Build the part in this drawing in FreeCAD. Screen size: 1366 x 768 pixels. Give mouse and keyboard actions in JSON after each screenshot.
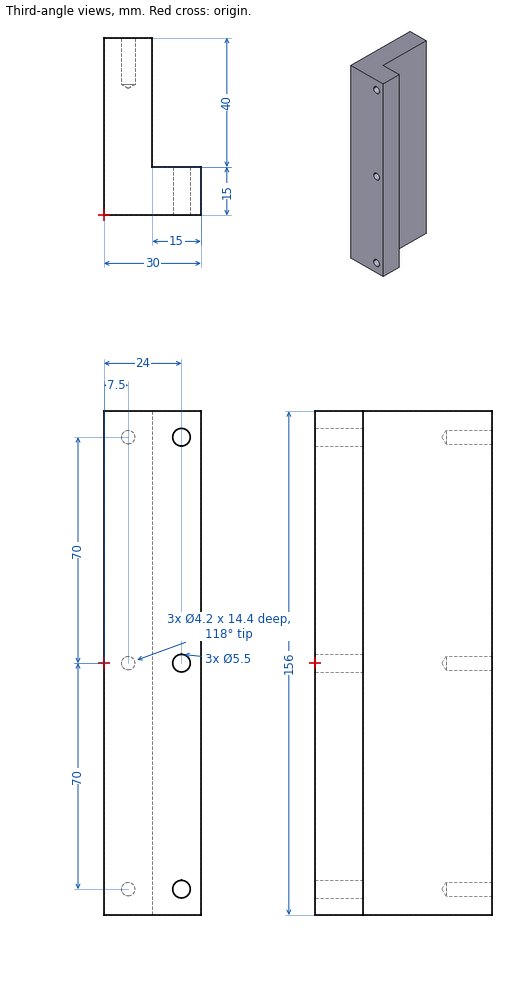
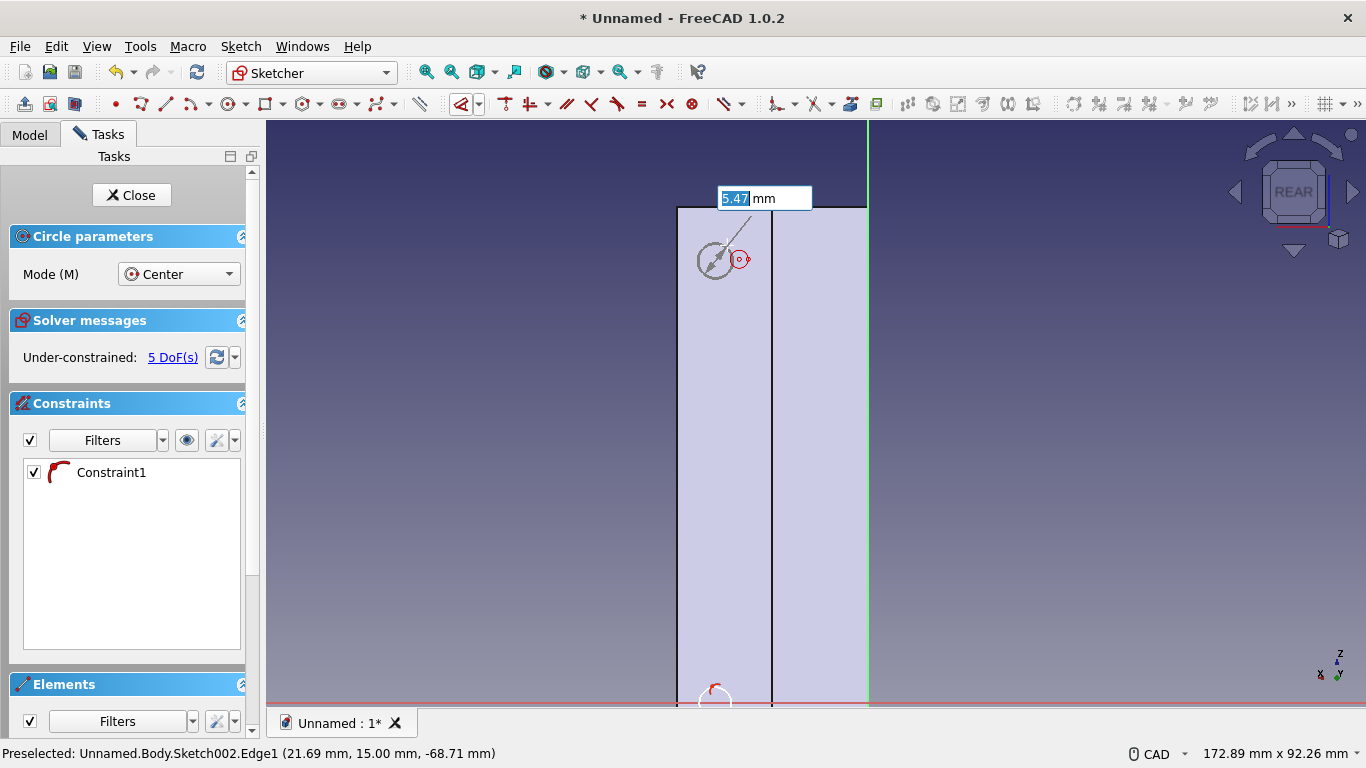
{"action": "left_click", "coordinate": [727, 246]}
{"action": "key", "text": "Escape"}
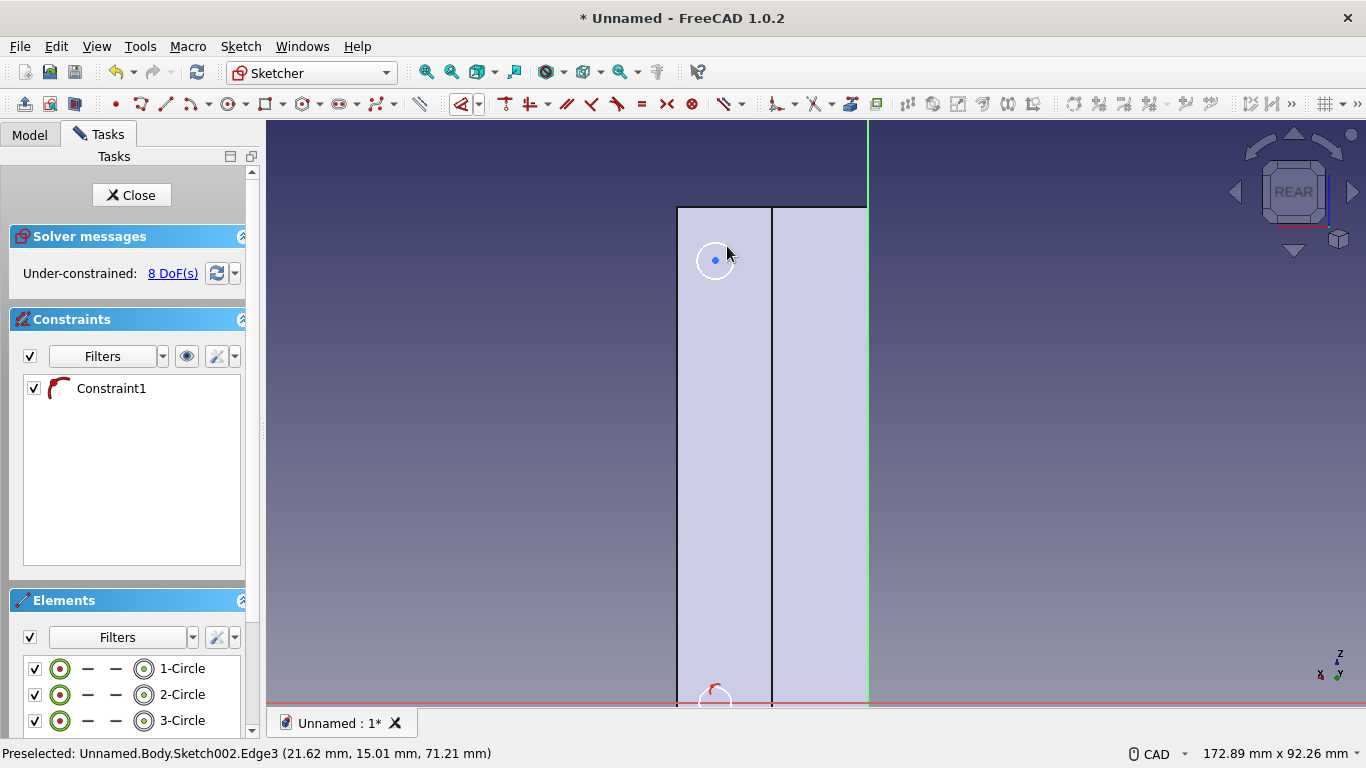
{"action": "scroll", "coordinate": [727, 245], "scroll_direction": "down", "scroll_amount": 5}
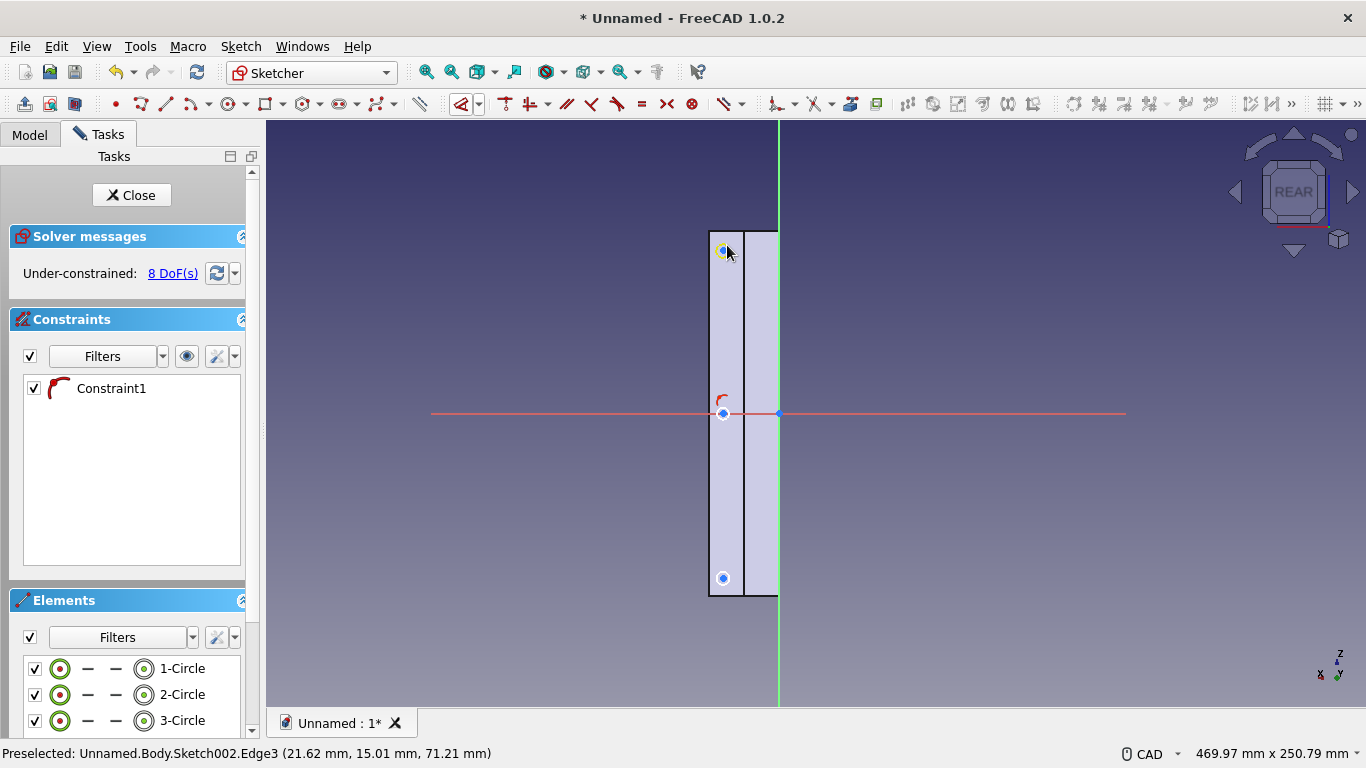
{"action": "scroll", "coordinate": [727, 410], "scroll_direction": "up", "scroll_amount": 6}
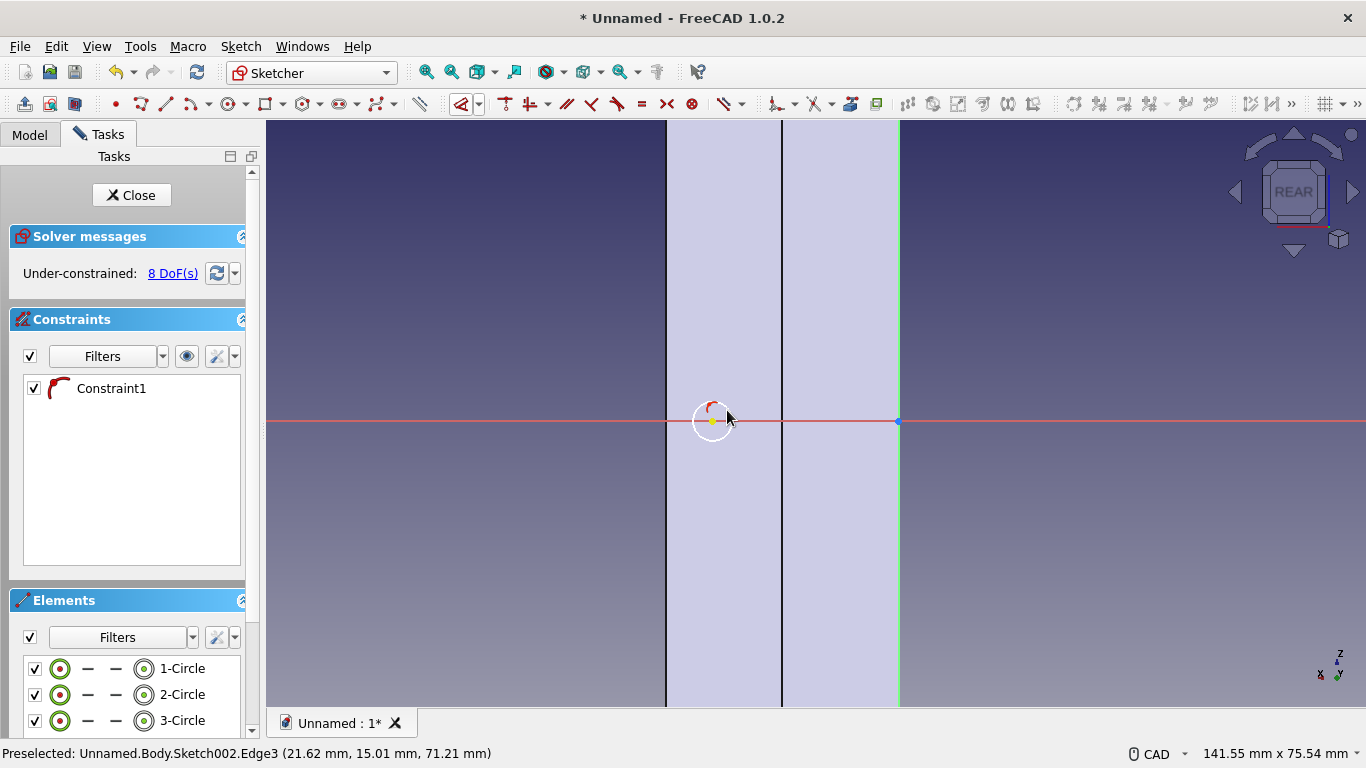
{"action": "left_click", "coordinate": [727, 407]}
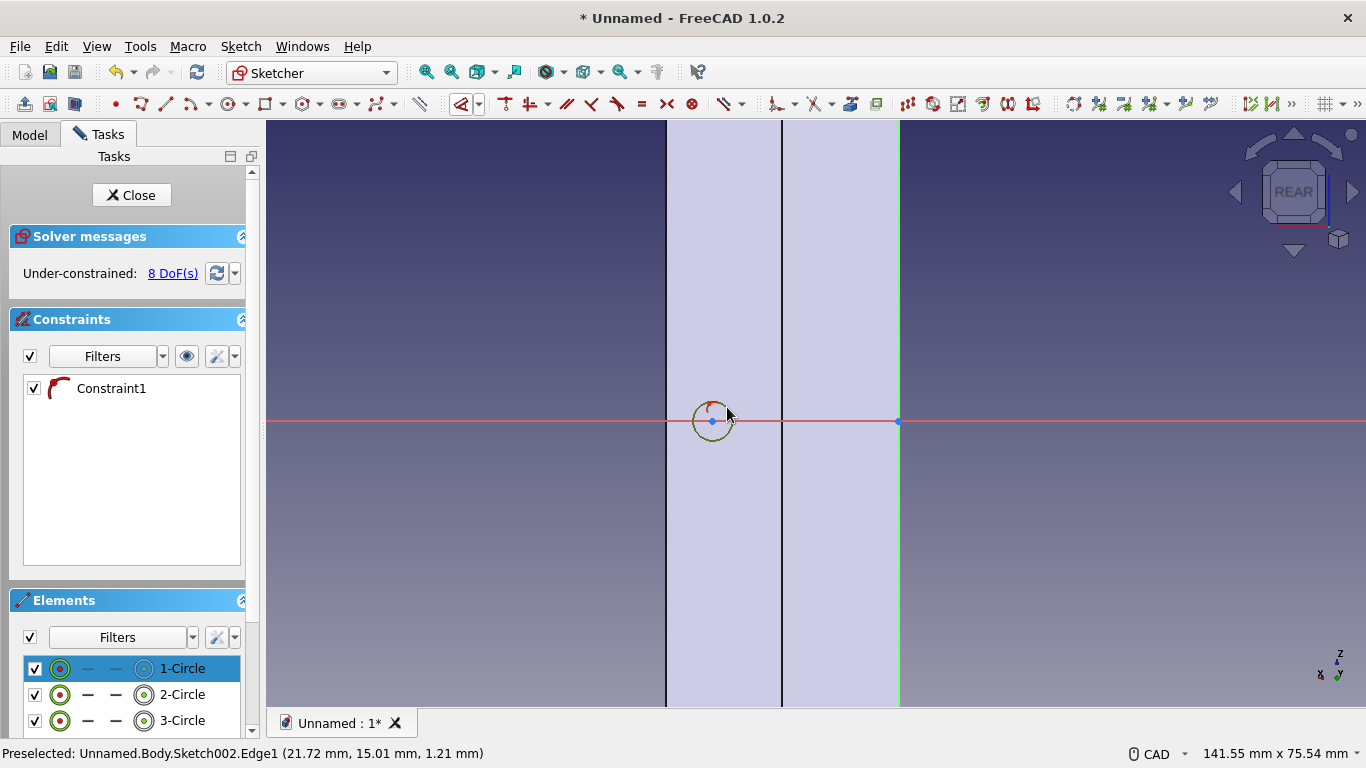
{"action": "scroll", "coordinate": [727, 410], "scroll_direction": "down", "scroll_amount": 6}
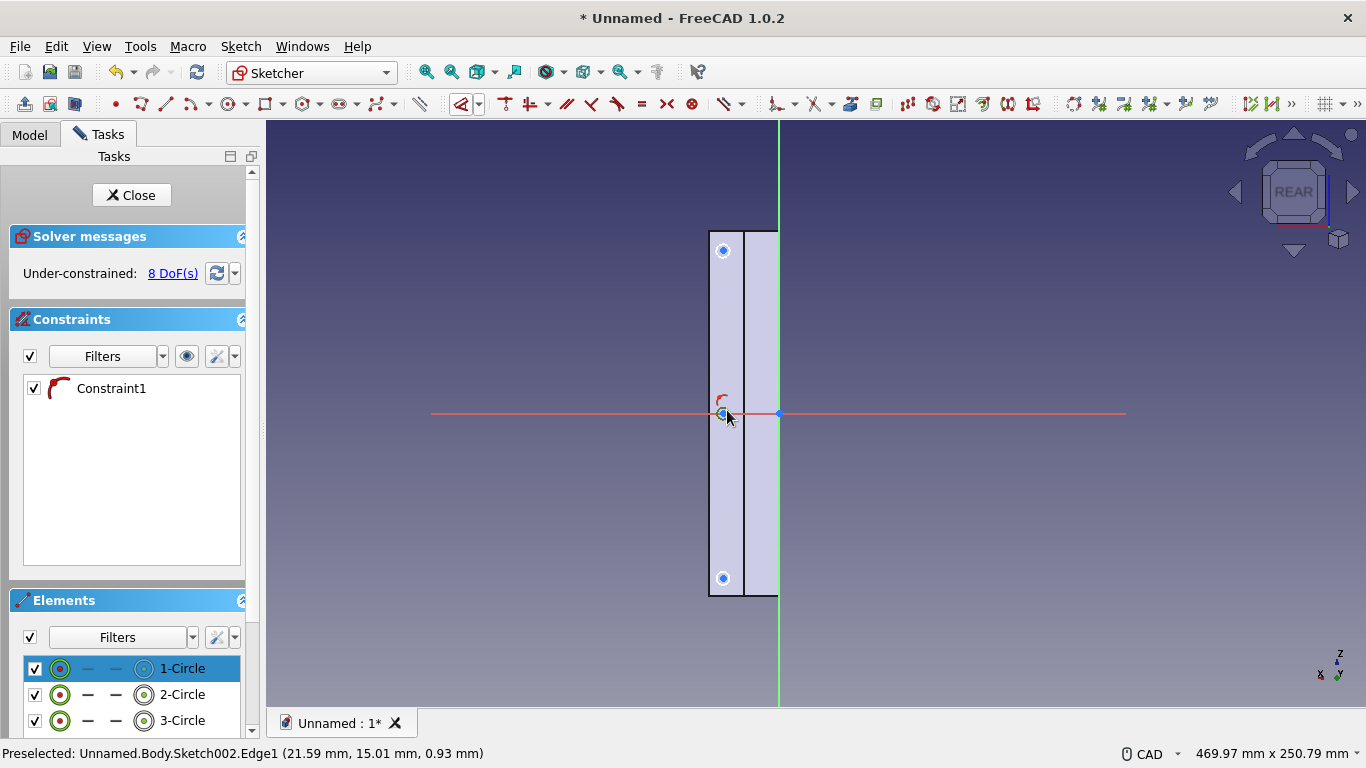
{"action": "scroll", "coordinate": [728, 574], "scroll_direction": "up", "scroll_amount": 4}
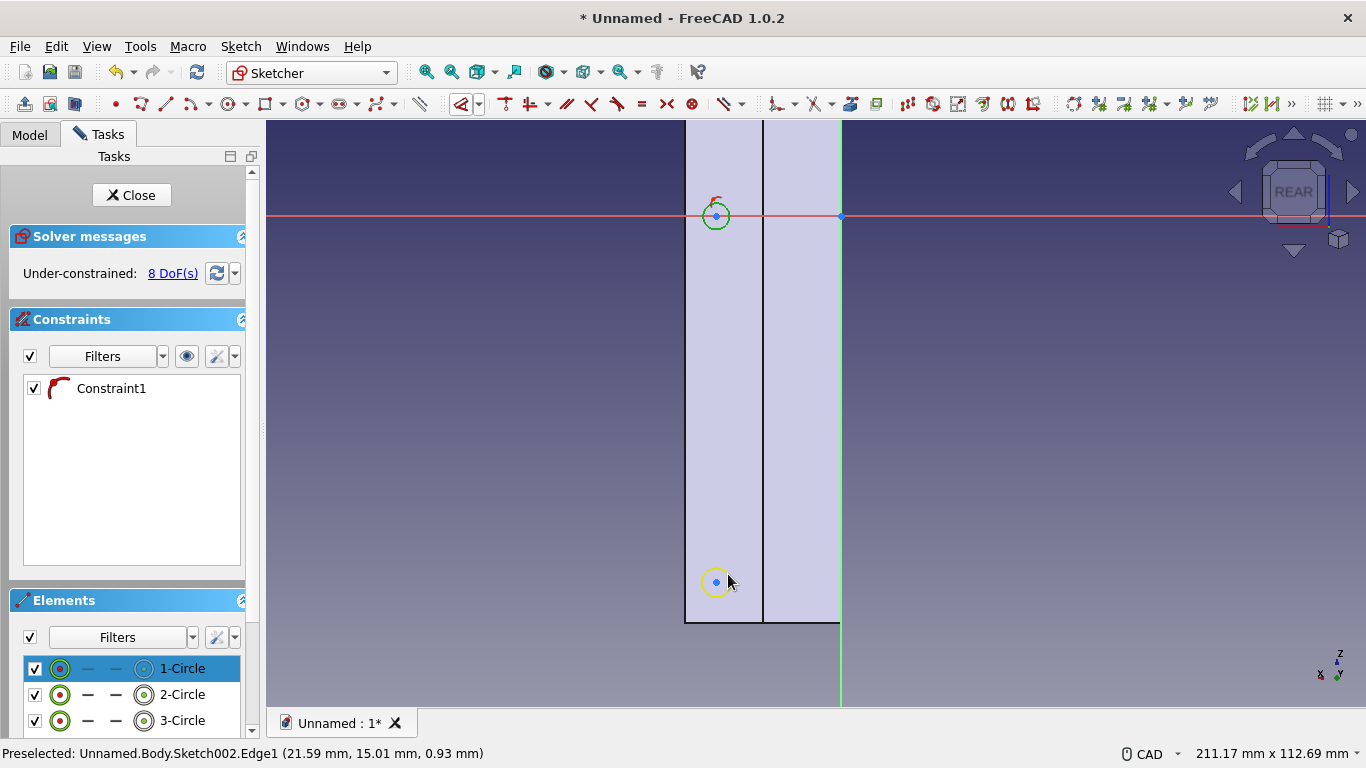
{"action": "left_click", "coordinate": [727, 573]}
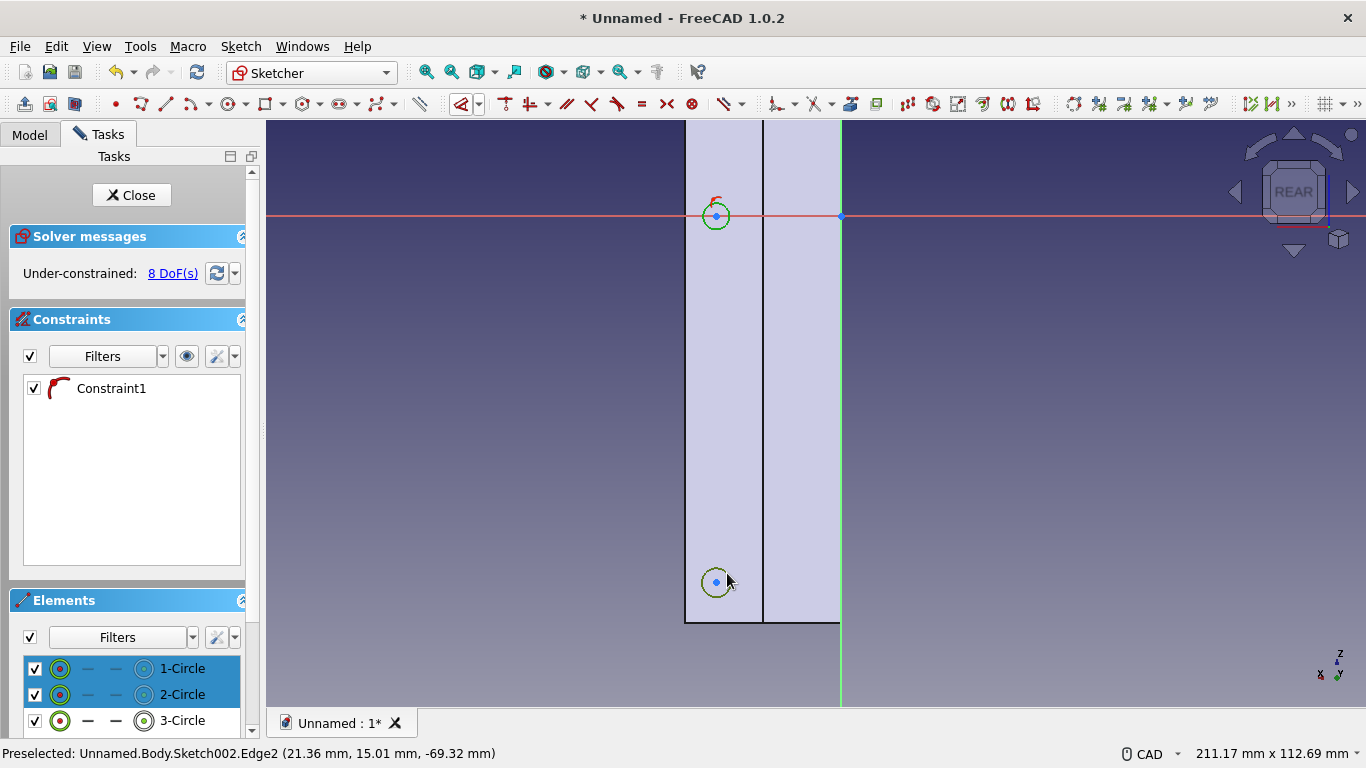
{"action": "scroll", "coordinate": [728, 574], "scroll_direction": "down", "scroll_amount": 4}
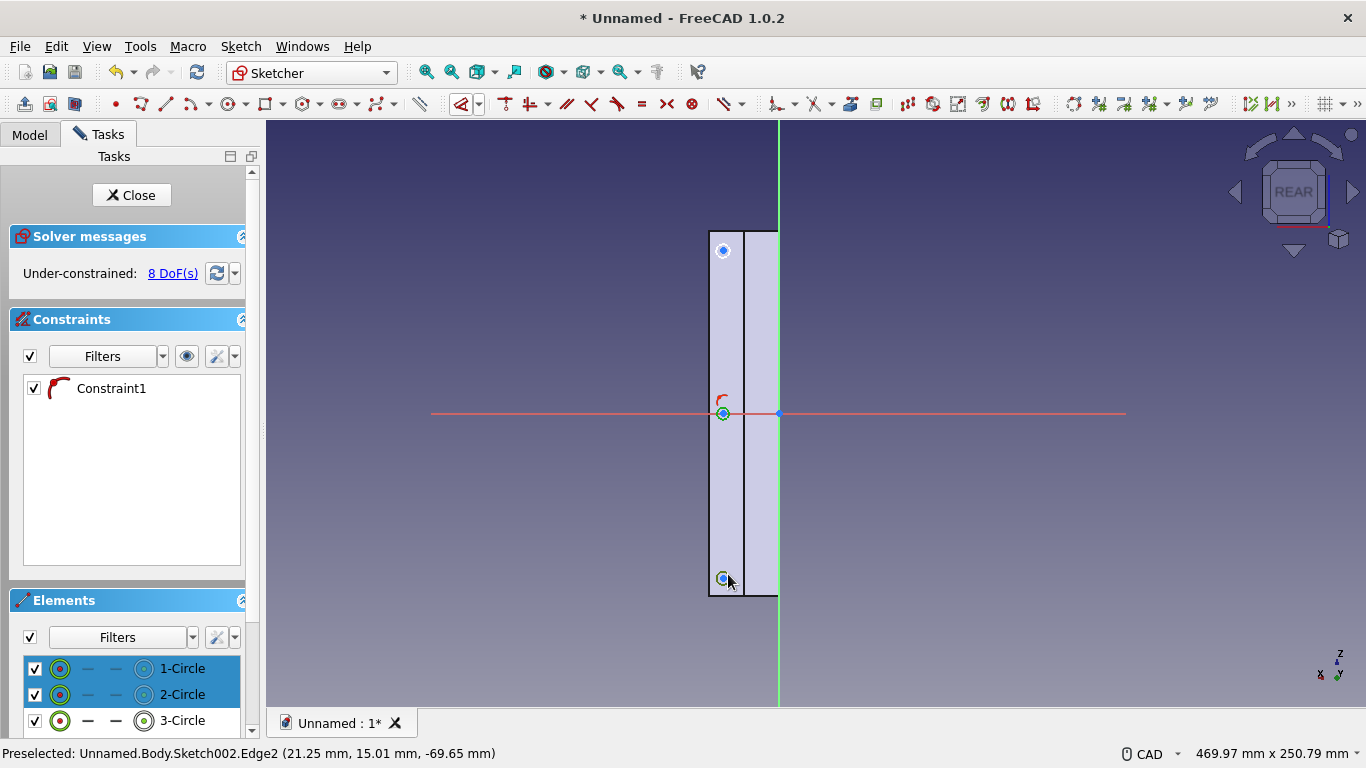
{"action": "scroll", "coordinate": [728, 246], "scroll_direction": "up", "scroll_amount": 4}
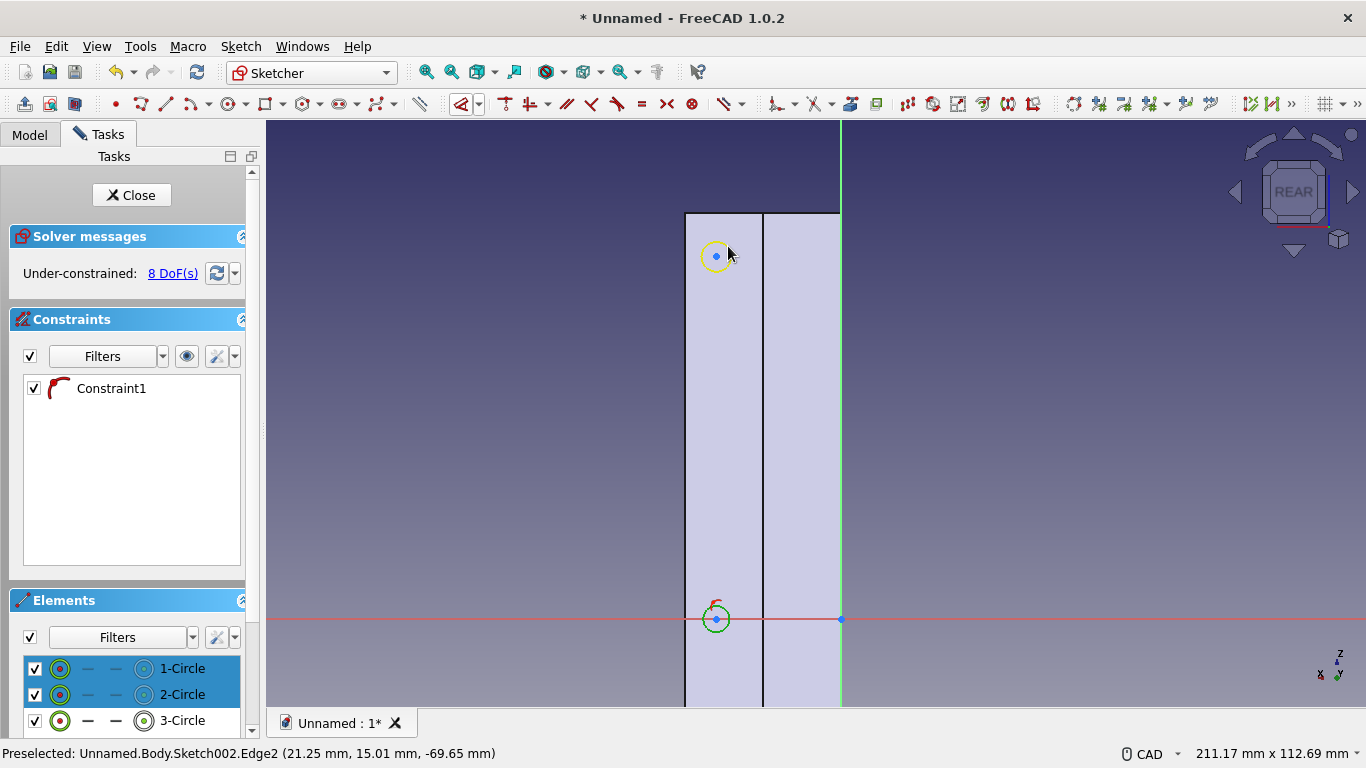
{"action": "left_click", "coordinate": [727, 246]}